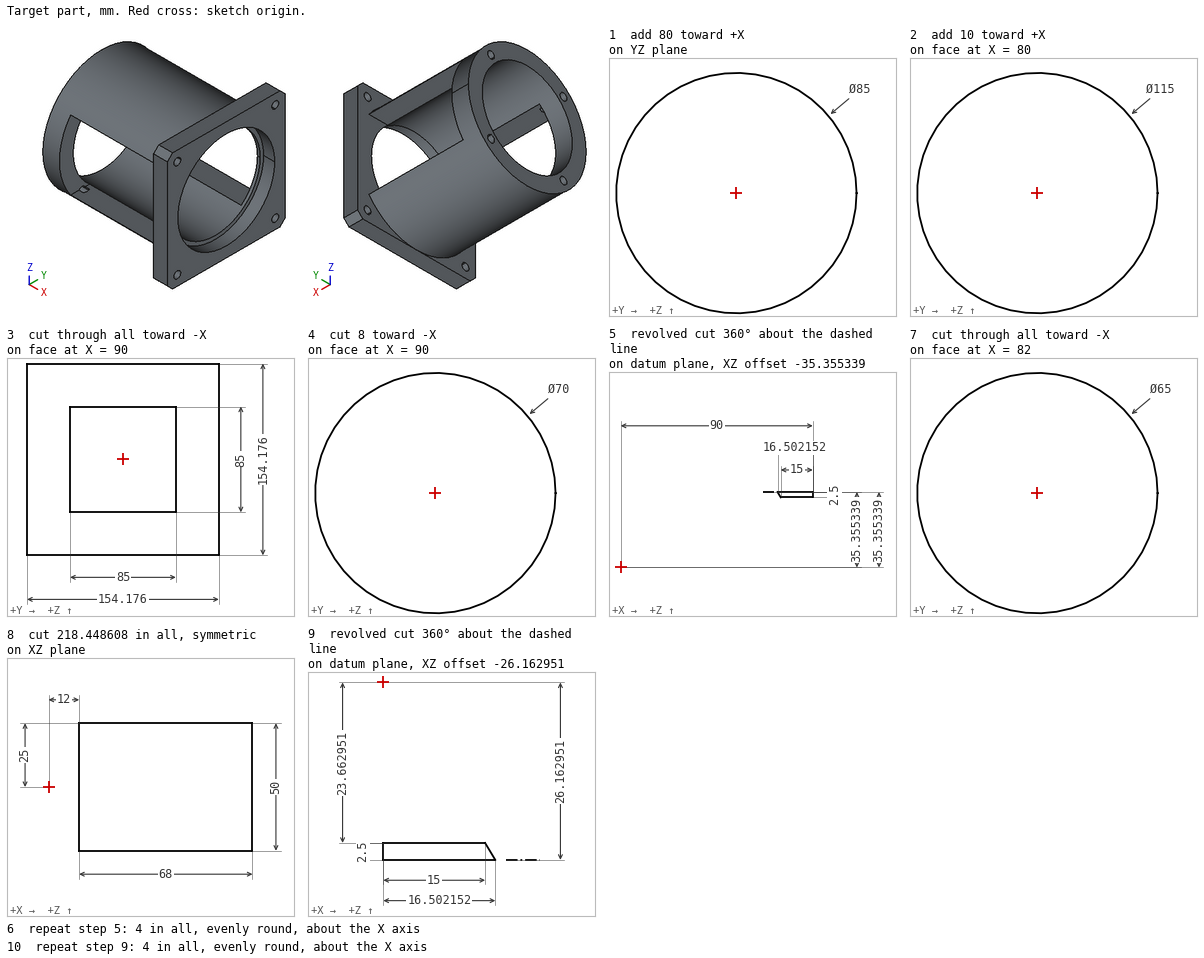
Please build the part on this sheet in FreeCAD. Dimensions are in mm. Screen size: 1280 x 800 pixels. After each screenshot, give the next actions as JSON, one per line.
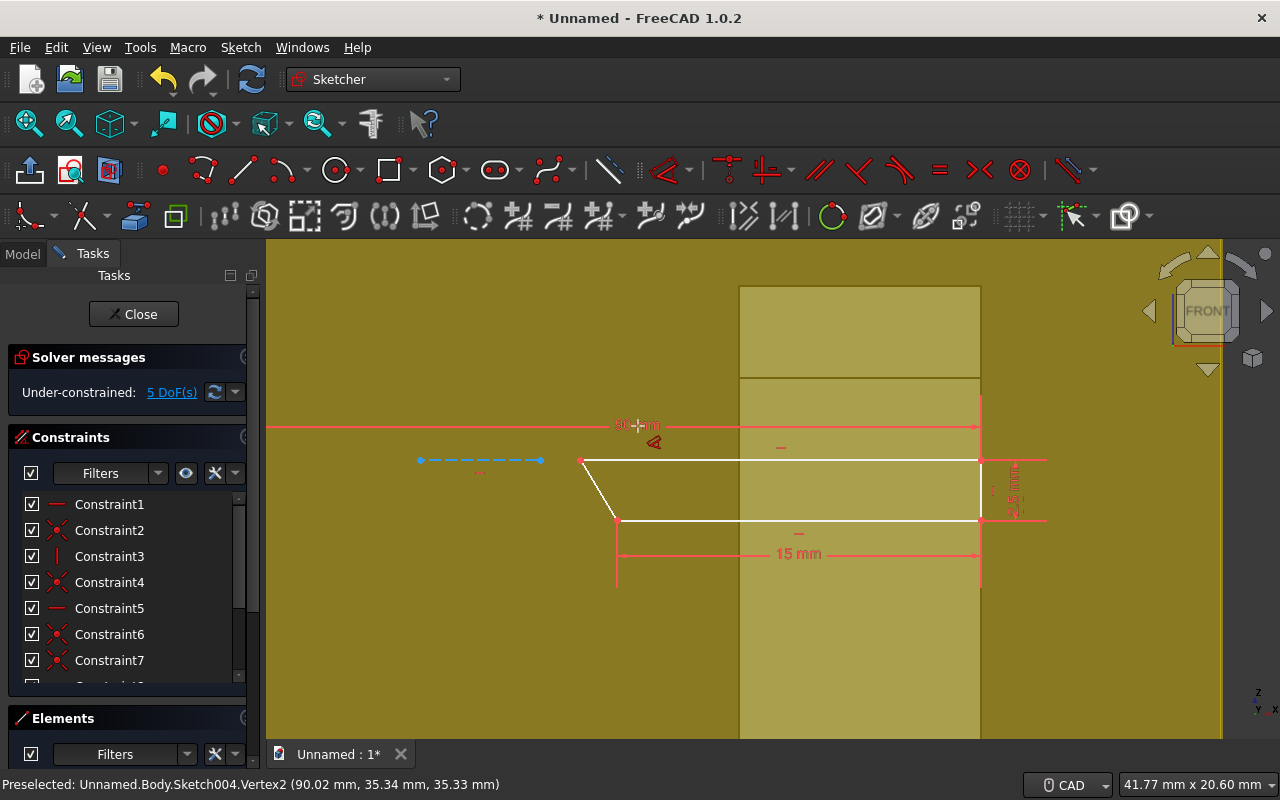
{"action": "left_click", "coordinate": [701, 460]}
{"action": "left_click", "coordinate": [781, 426]}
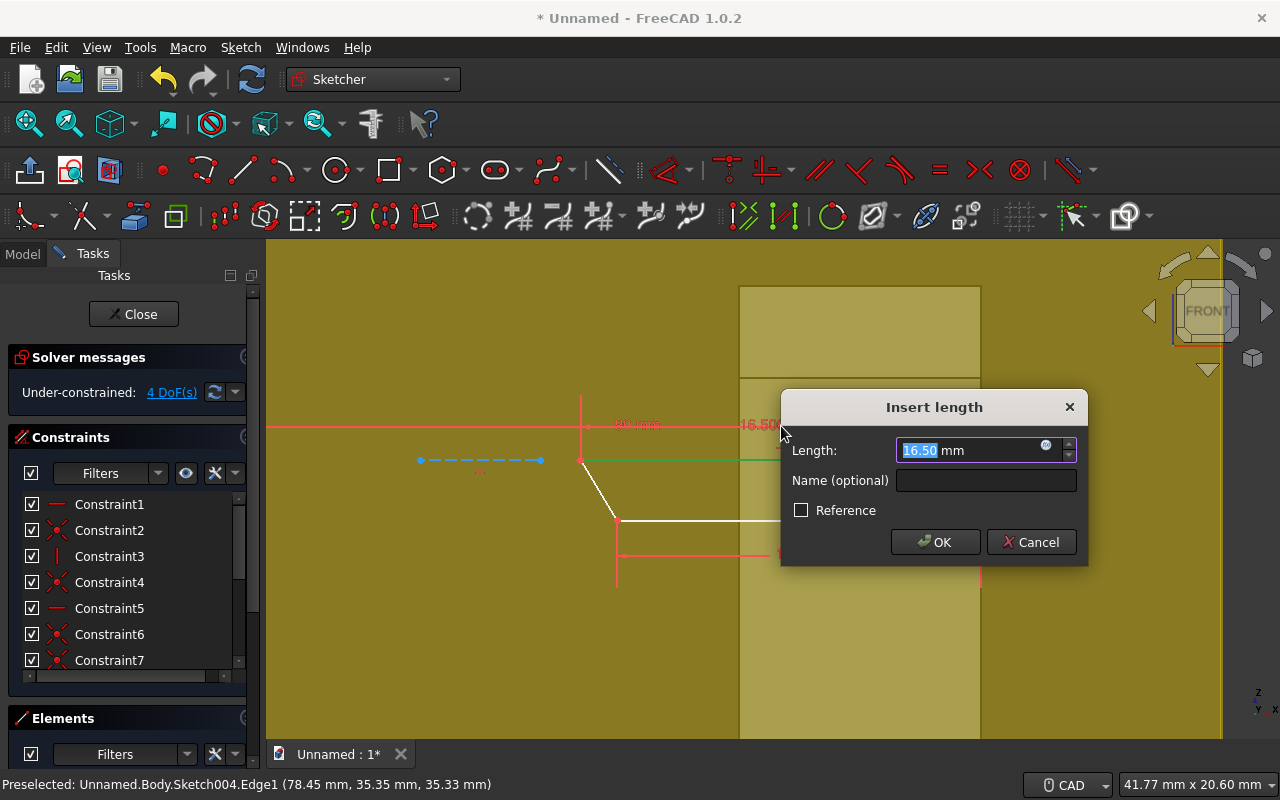
{"action": "type", "text": "16.502152"}
{"action": "key", "text": "Return"}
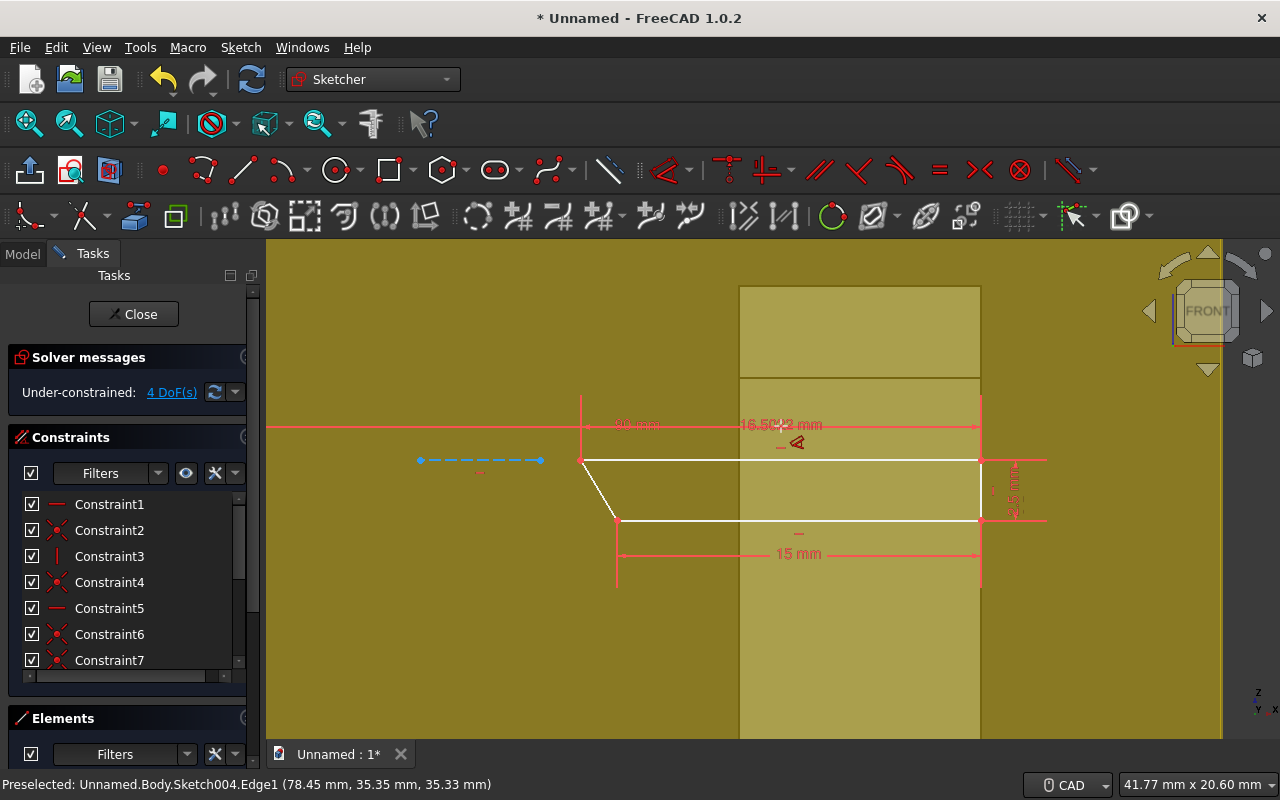
{"action": "left_click", "coordinate": [581, 460]}
{"action": "left_click", "coordinate": [615, 586]}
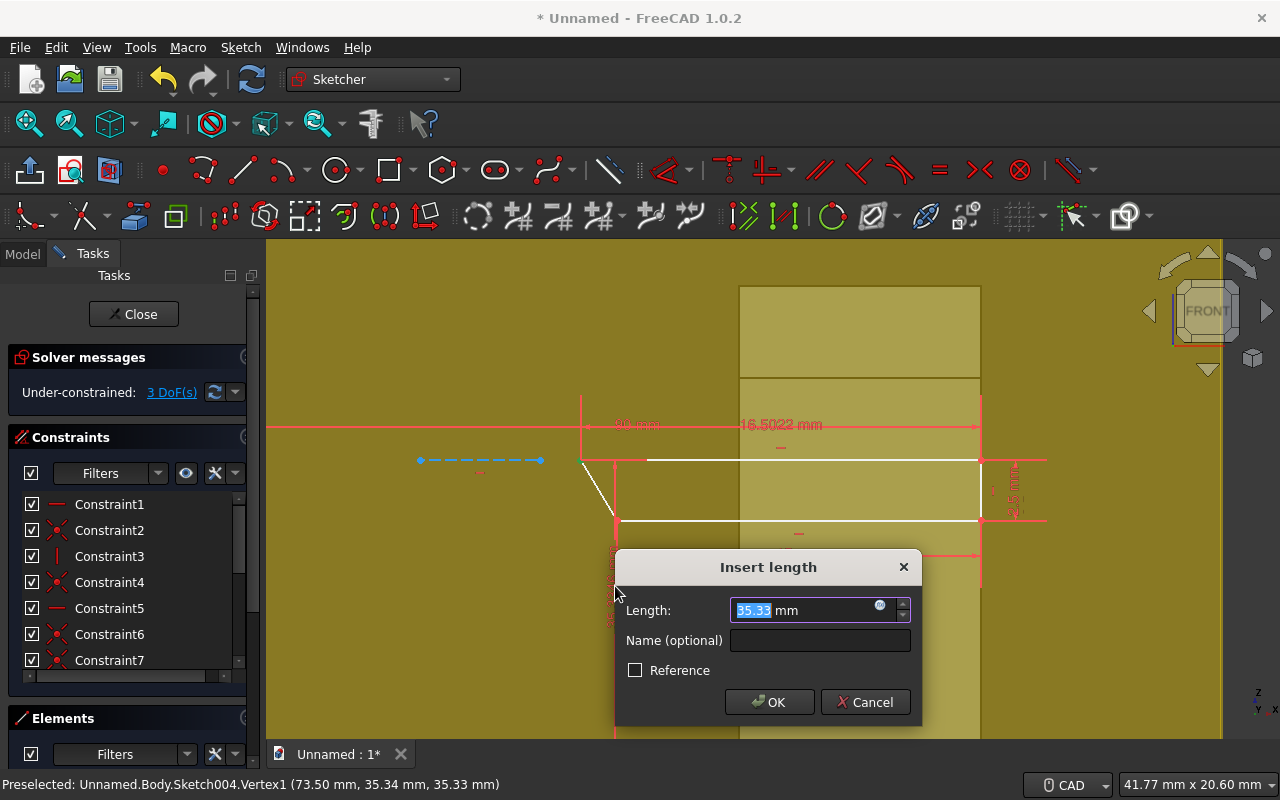
{"action": "type", "text": "35.355339"}
{"action": "key", "text": "Return"}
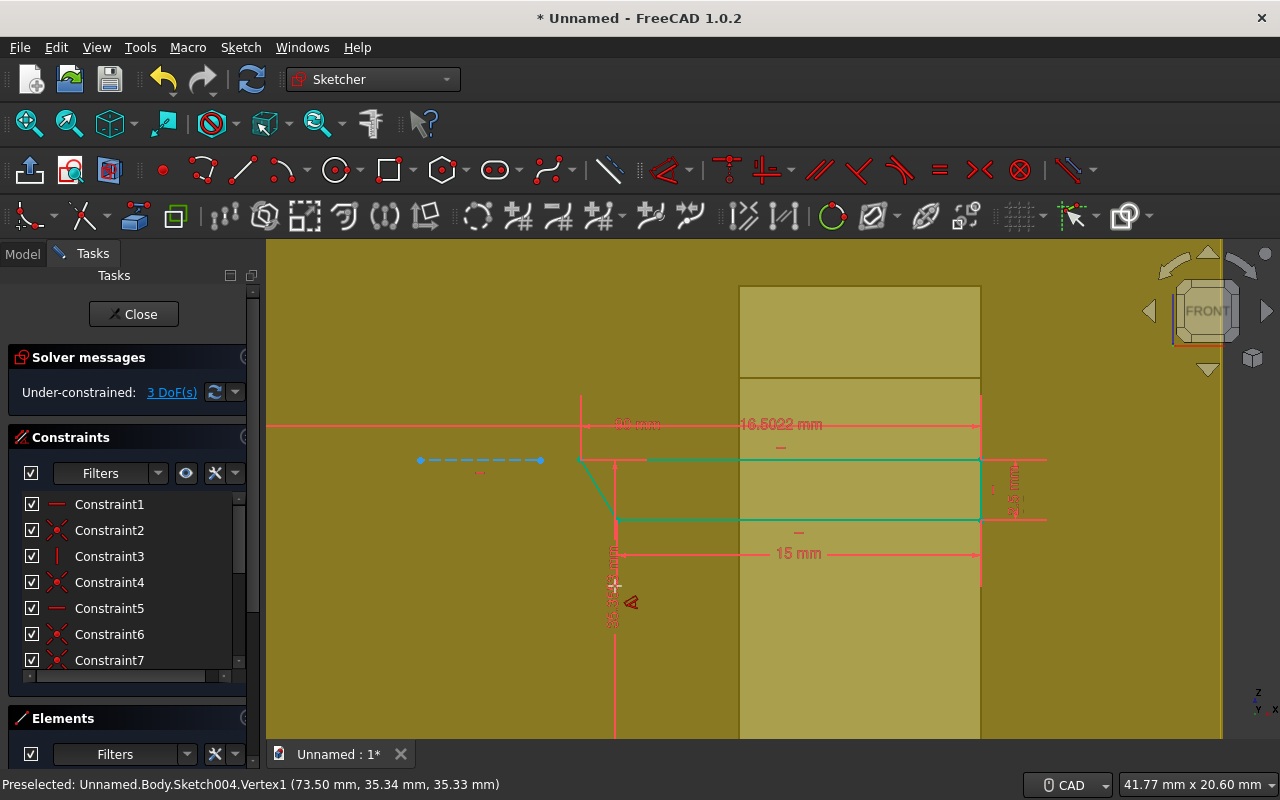
{"action": "left_click", "coordinate": [541, 460]}
{"action": "left_click", "coordinate": [575, 528]}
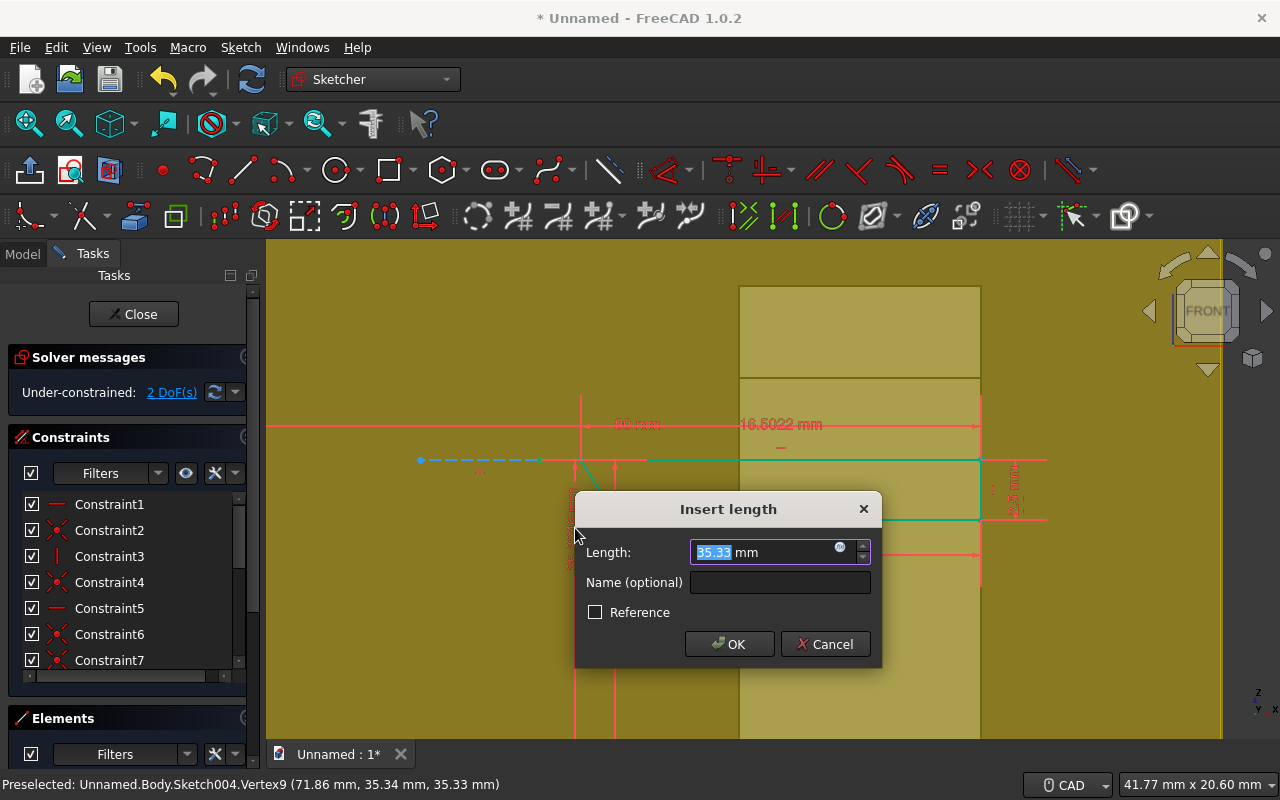
{"action": "type", "text": "35.355339"}
{"action": "key", "text": "Return"}
{"action": "key", "text": "Escape"}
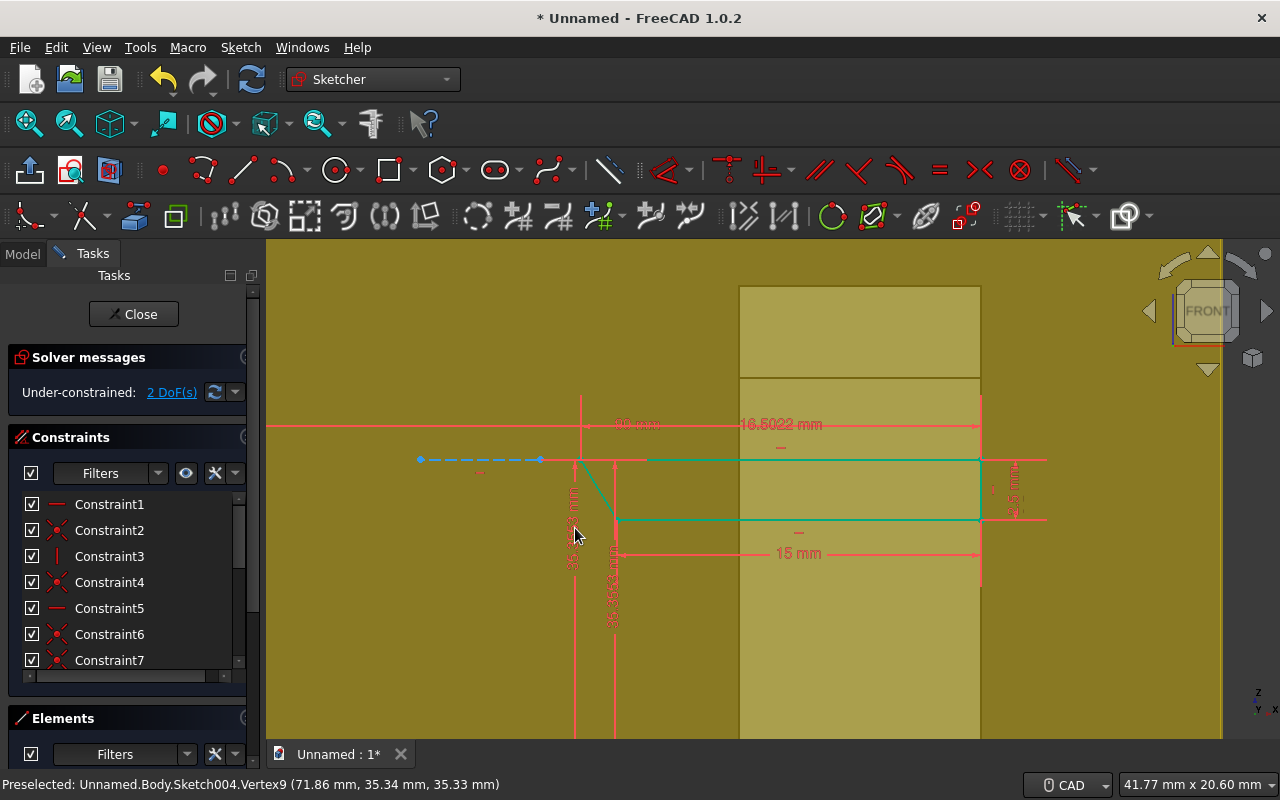
{"action": "left_click", "coordinate": [134, 314]}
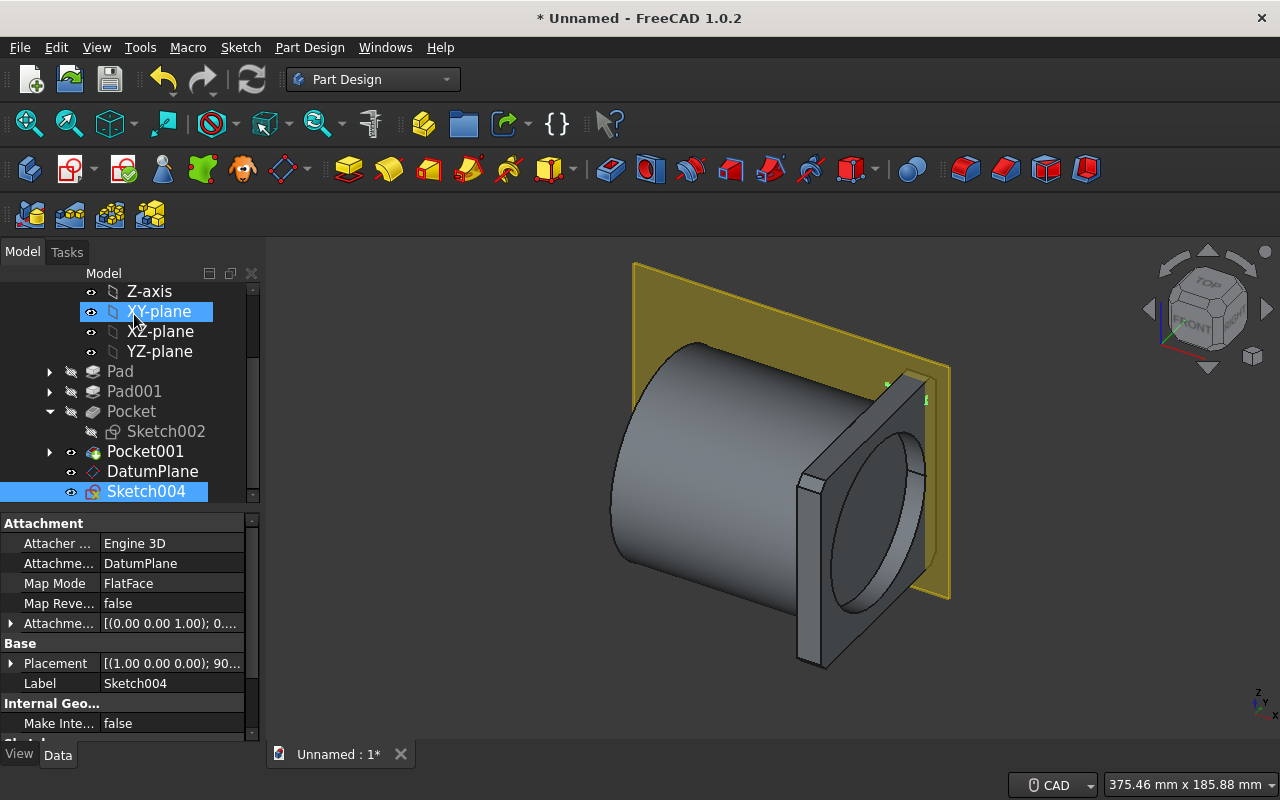
{"action": "left_click", "coordinate": [692, 170]}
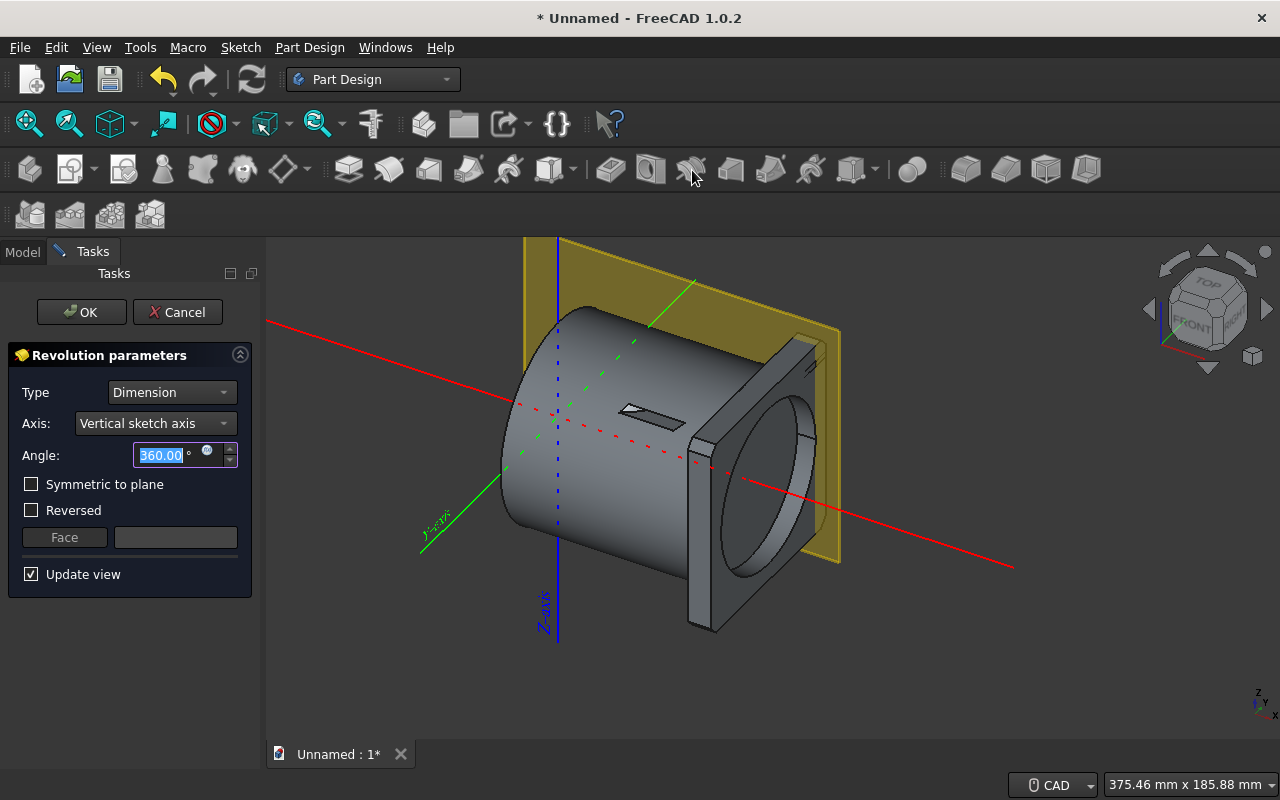
{"action": "left_click", "coordinate": [156, 424]}